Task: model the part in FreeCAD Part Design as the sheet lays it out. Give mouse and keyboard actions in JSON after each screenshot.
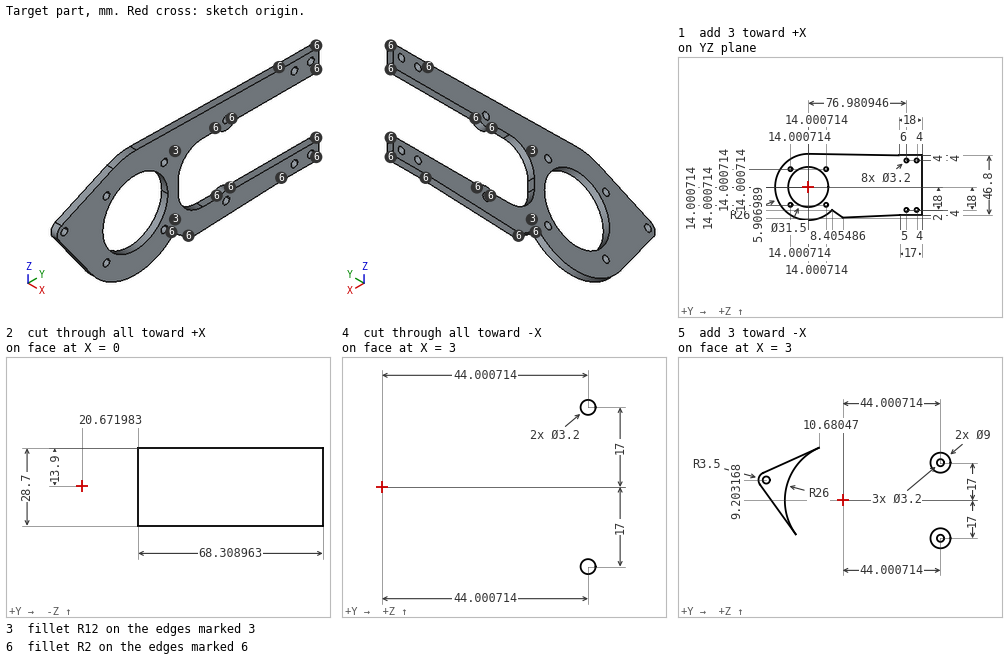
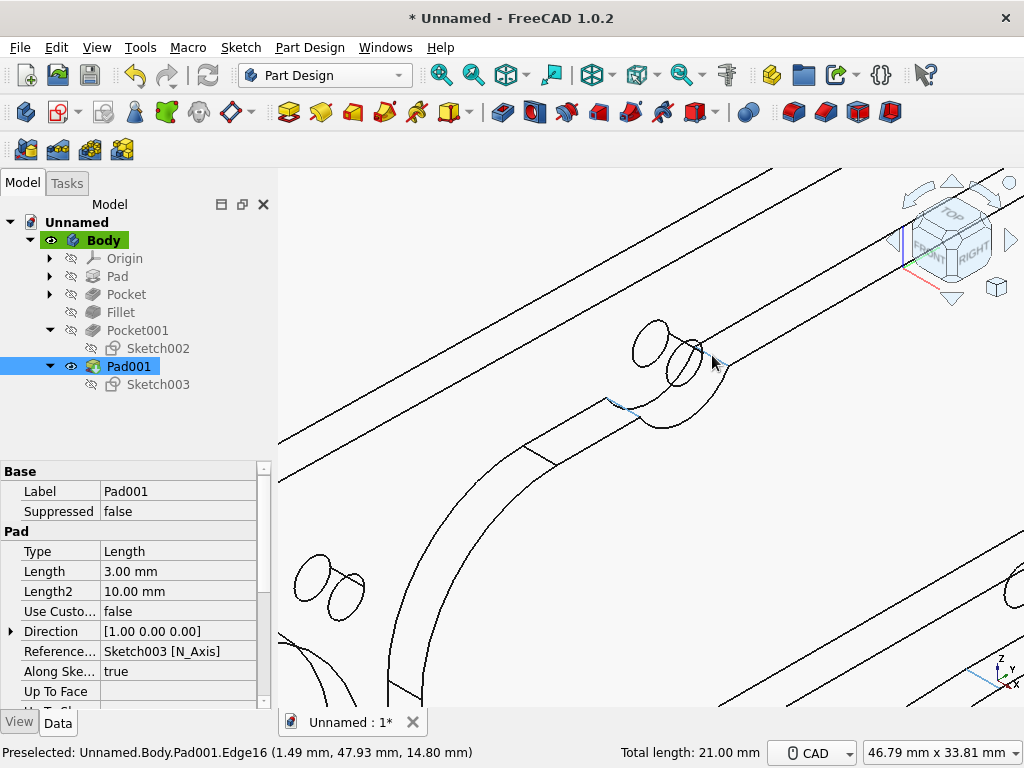
{"action": "left_click", "coordinate": [442, 76]}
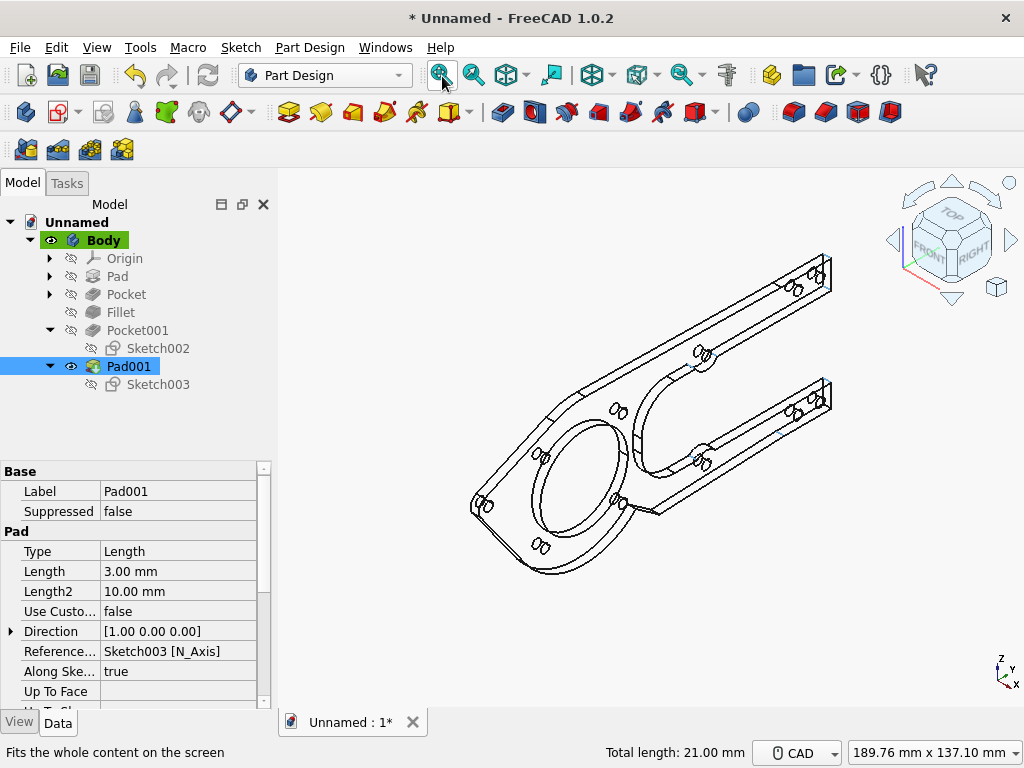
{"action": "key", "text": "2"}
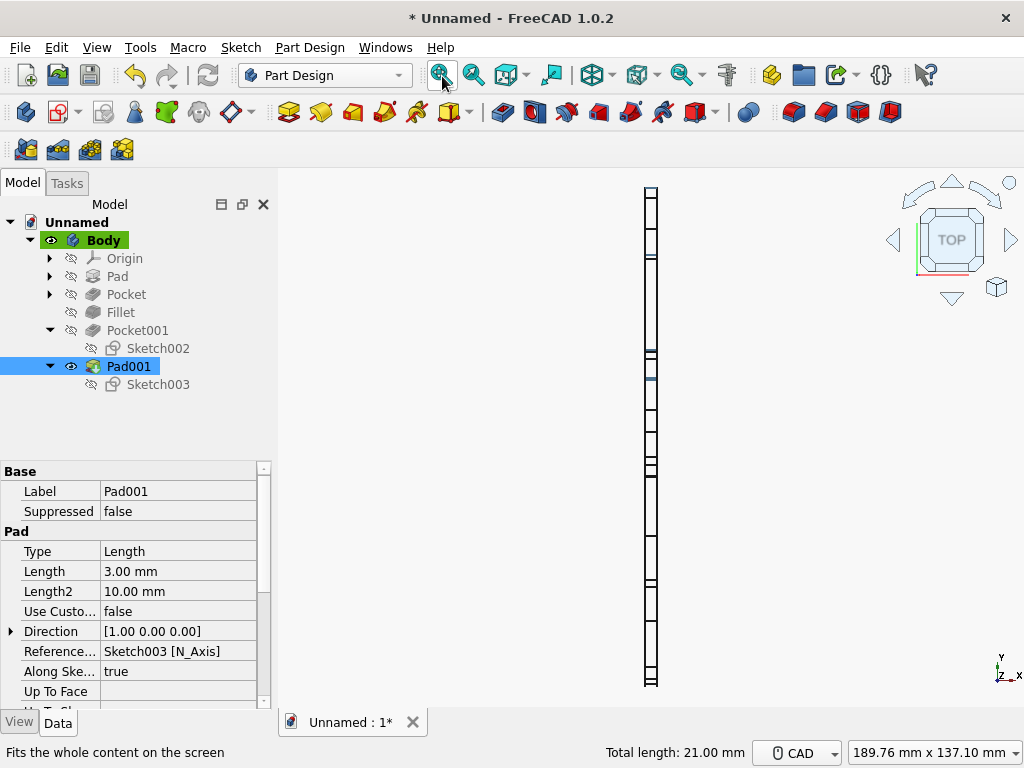
{"action": "scroll", "coordinate": [651, 258], "scroll_direction": "up", "scroll_amount": 7}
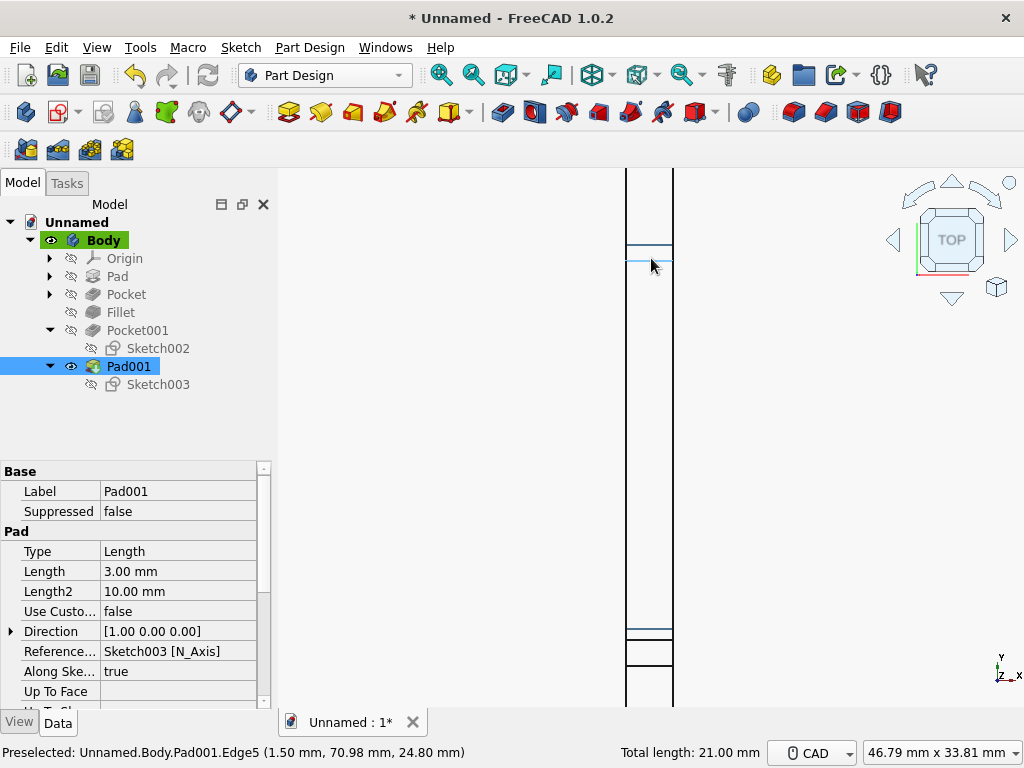
{"action": "left_click", "coordinate": [649, 260], "text": "ctrl"}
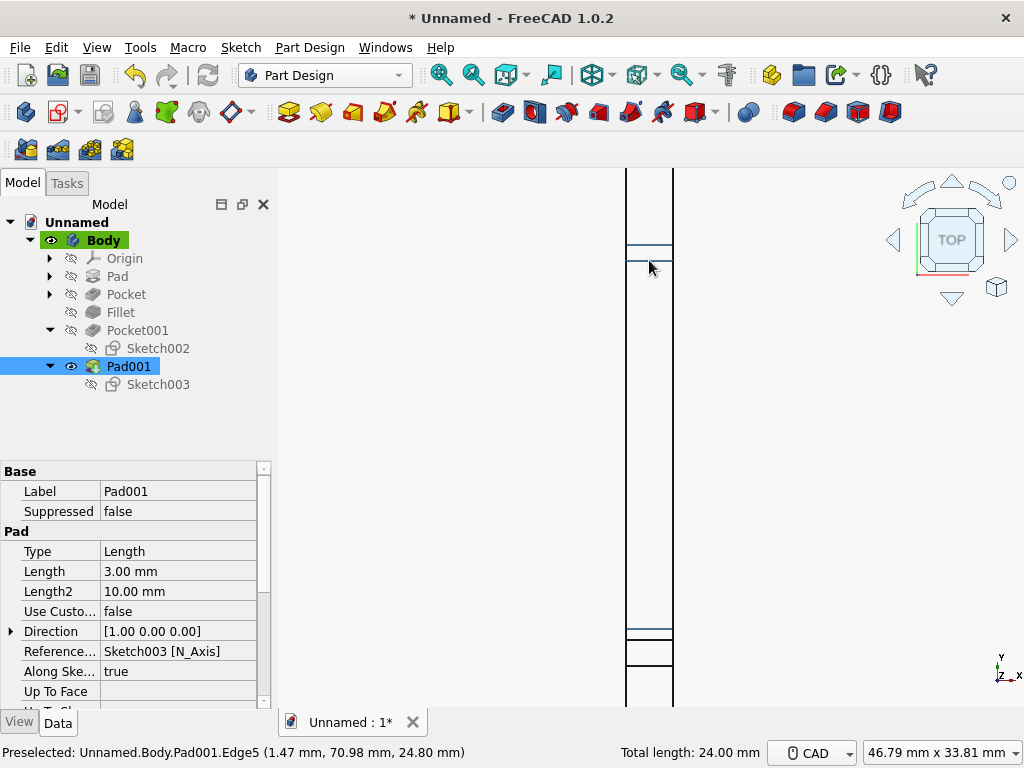
{"action": "left_click", "coordinate": [649, 639], "text": "ctrl"}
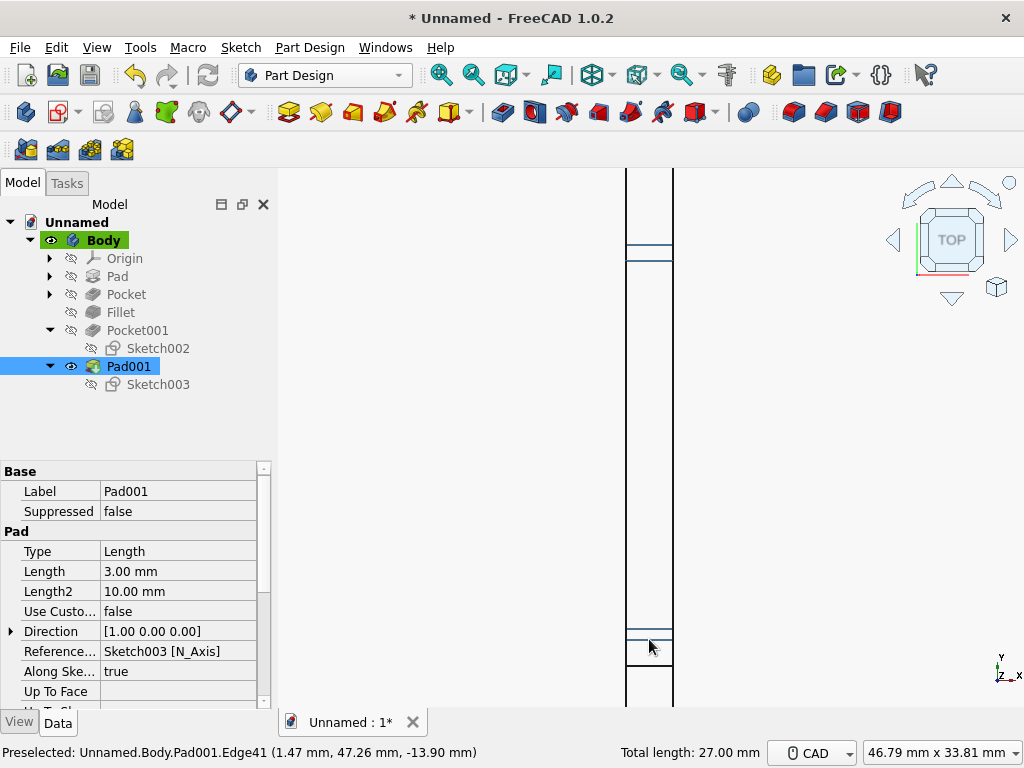
{"action": "left_click", "coordinate": [442, 76]}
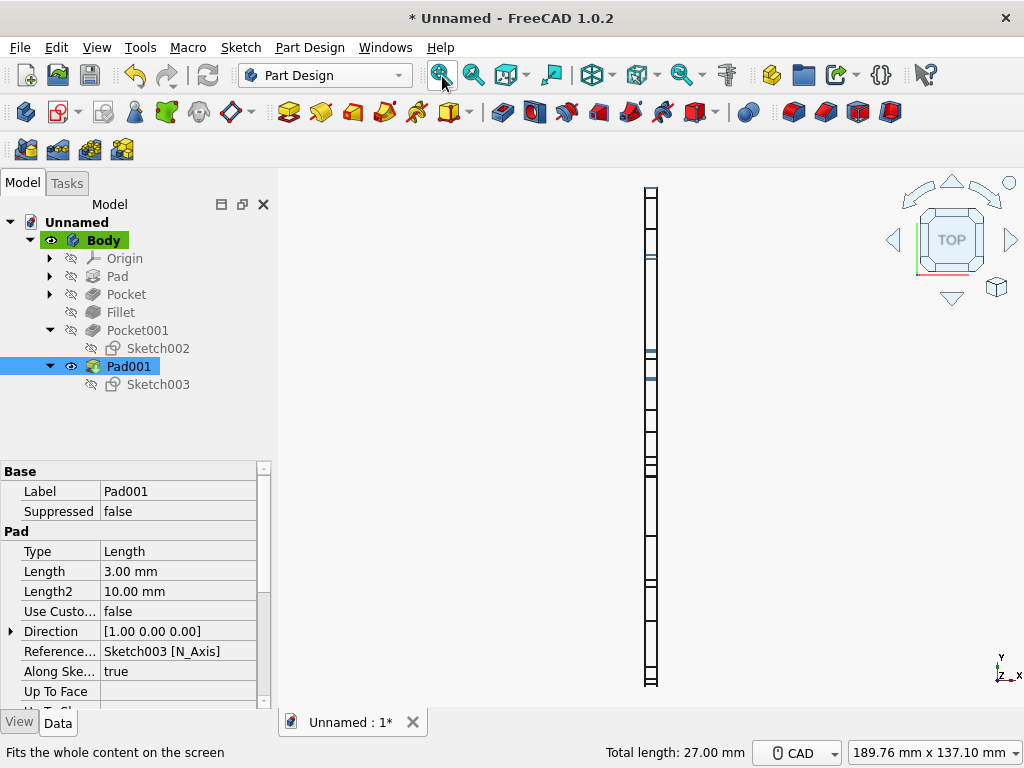
{"action": "key", "text": "1"}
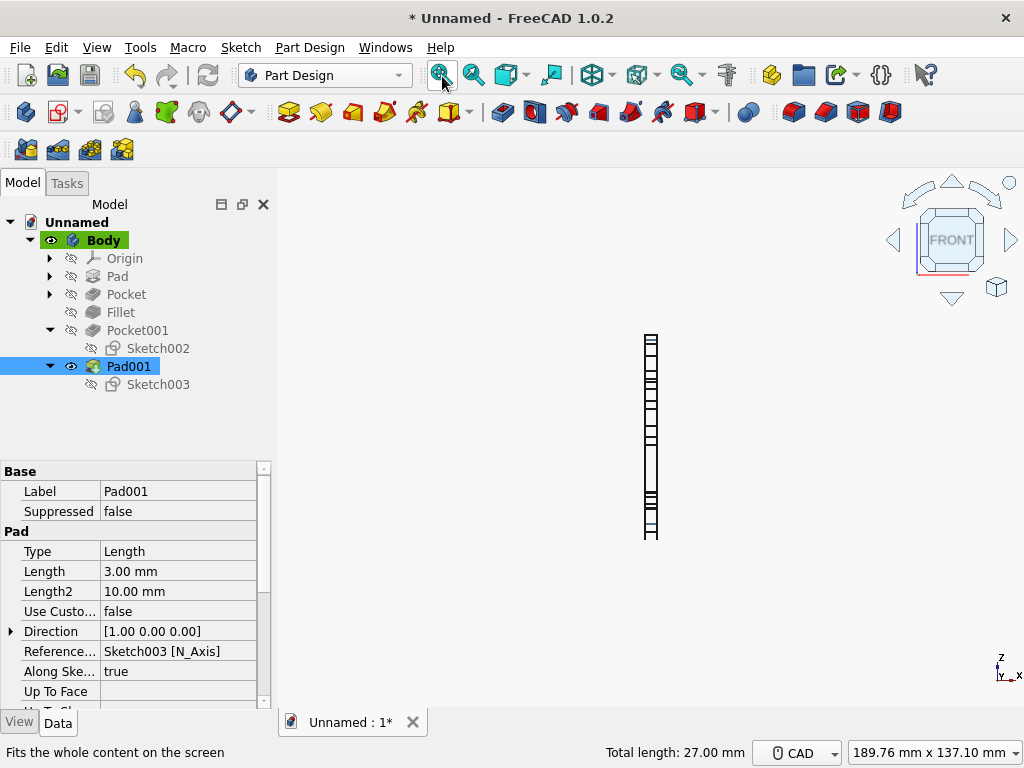
{"action": "left_click", "coordinate": [442, 76]}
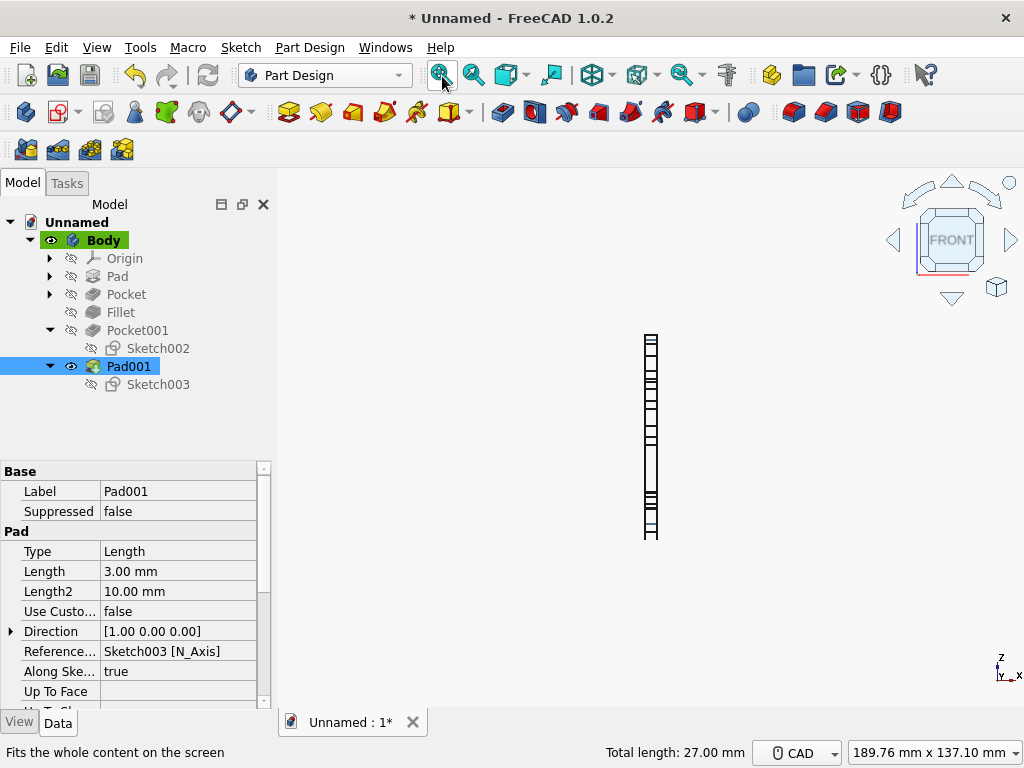
{"action": "scroll", "coordinate": [651, 523], "scroll_direction": "up", "scroll_amount": 7}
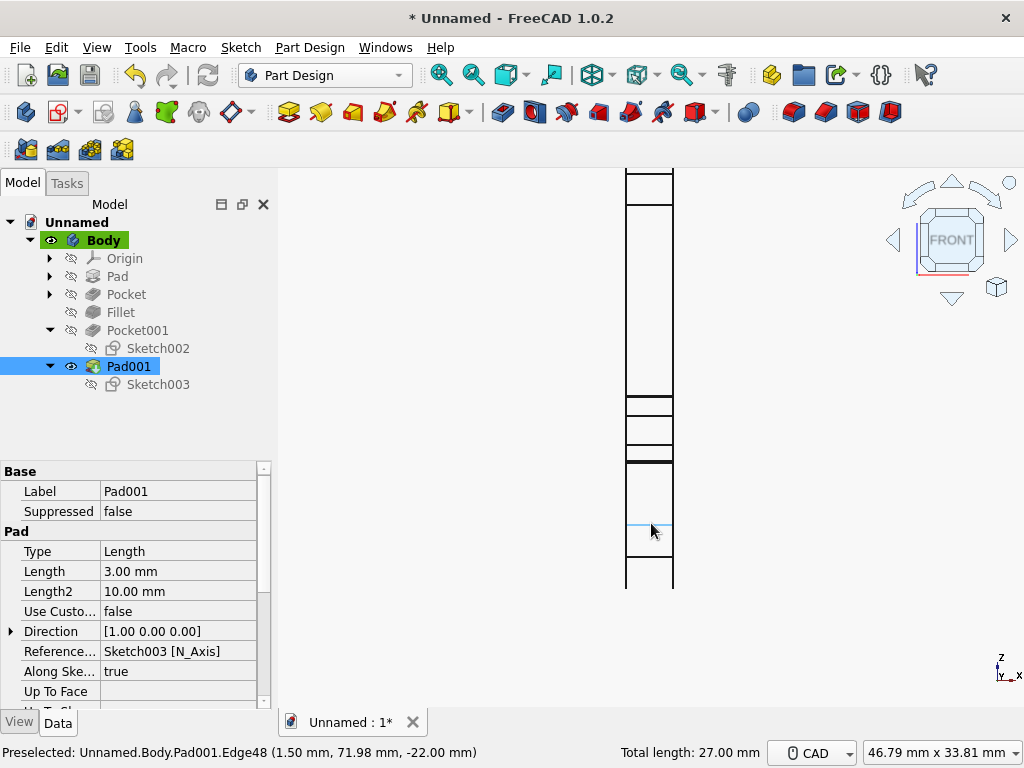
{"action": "left_click", "coordinate": [649, 556], "text": "ctrl"}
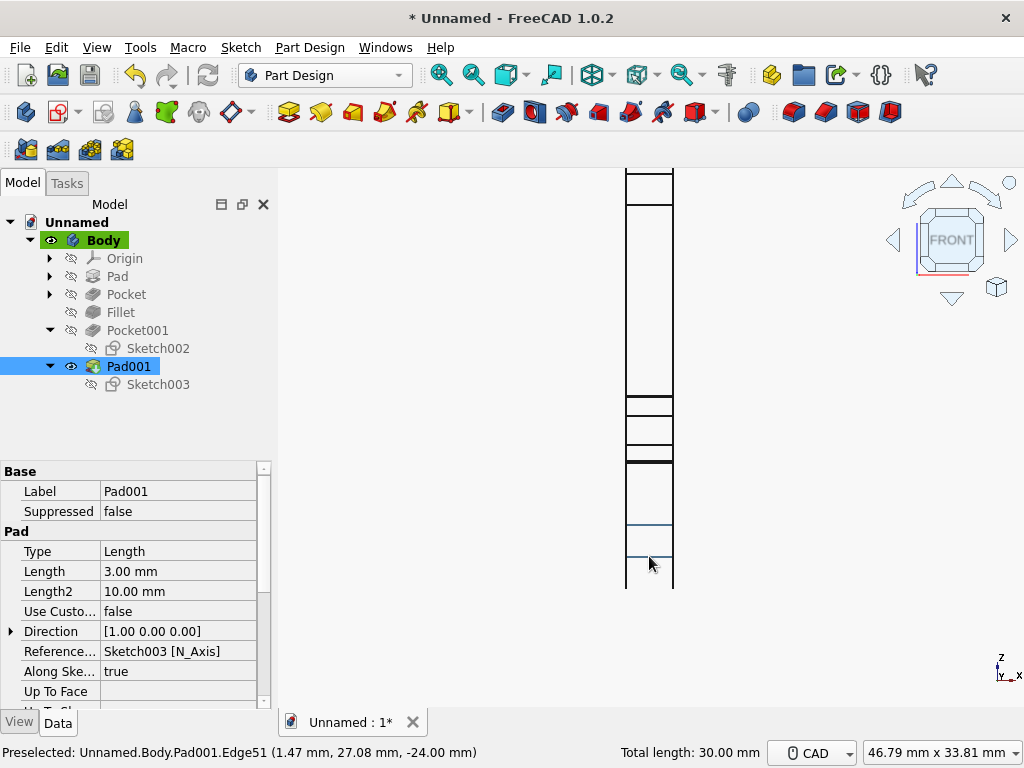
{"action": "left_click", "coordinate": [649, 462], "text": "ctrl"}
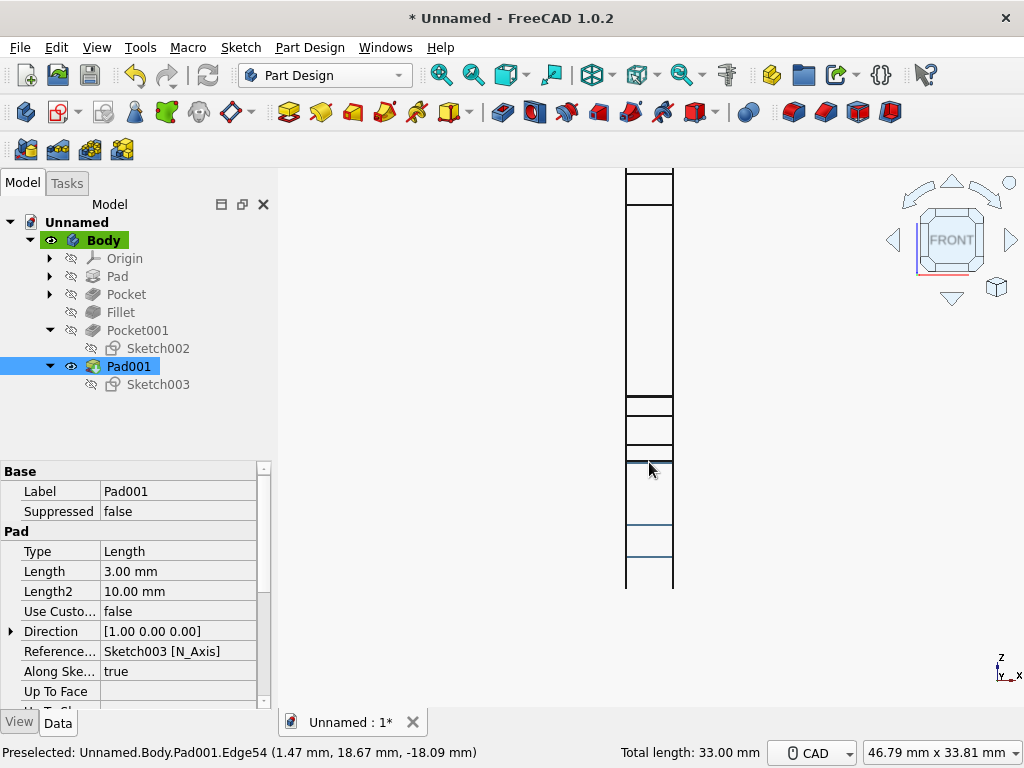
{"action": "left_click", "coordinate": [442, 76]}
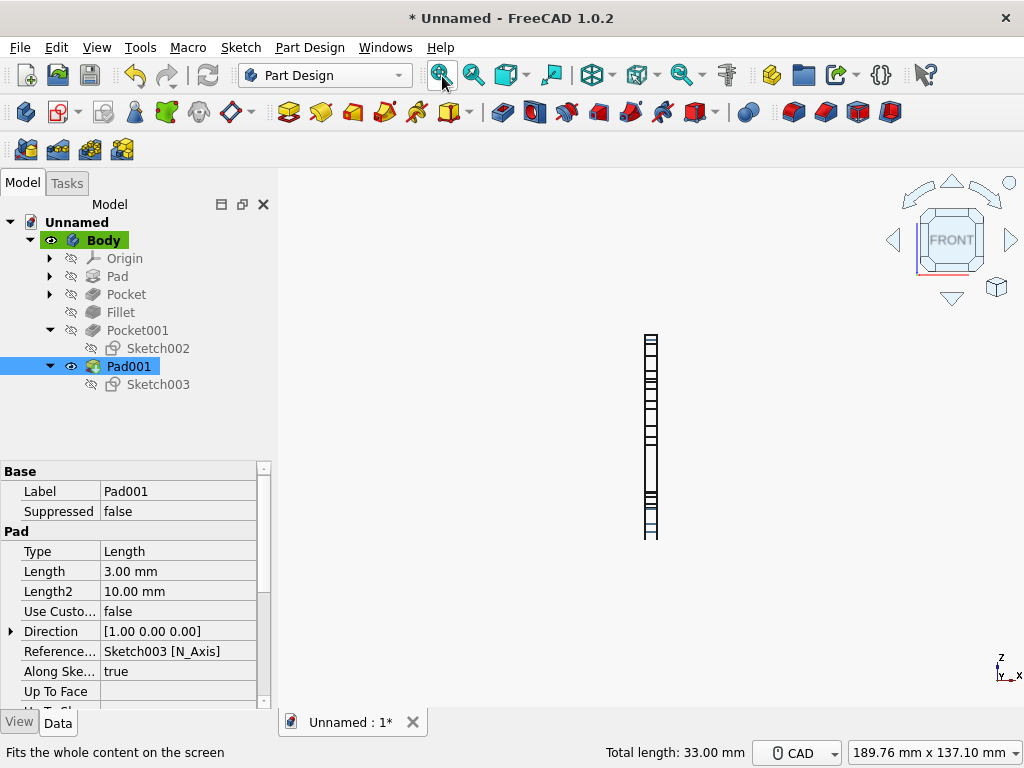
{"action": "key", "text": "3"}